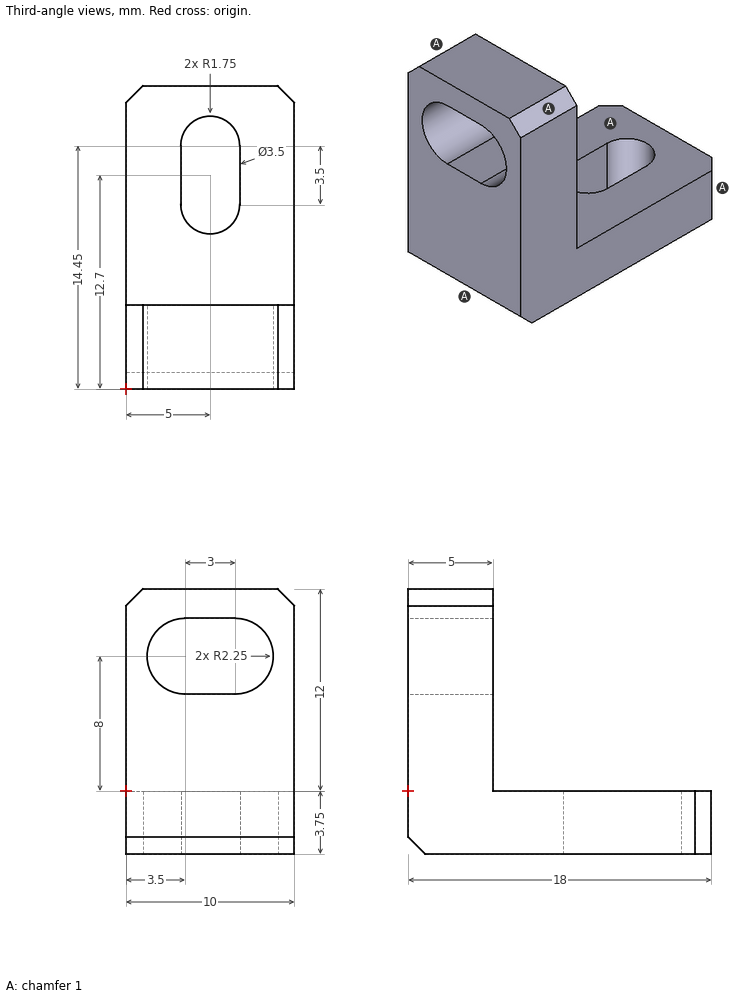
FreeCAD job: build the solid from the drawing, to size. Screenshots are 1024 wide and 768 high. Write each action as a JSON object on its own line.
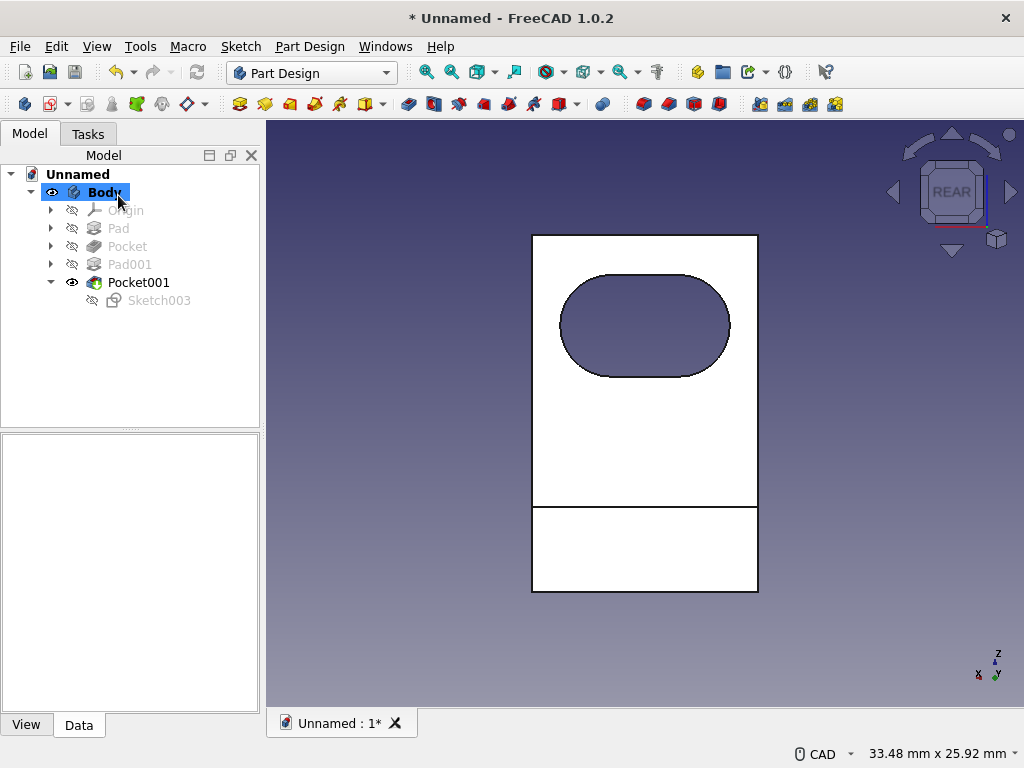
{"action": "left_click", "coordinate": [758, 548]}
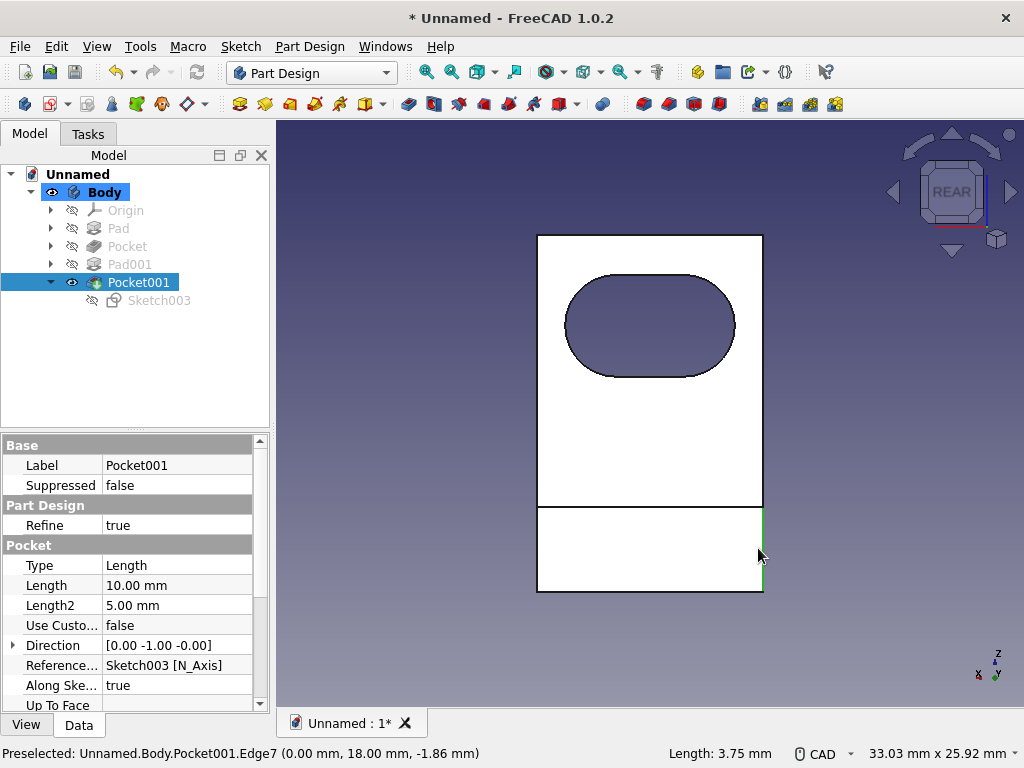
{"action": "key", "text": "0"}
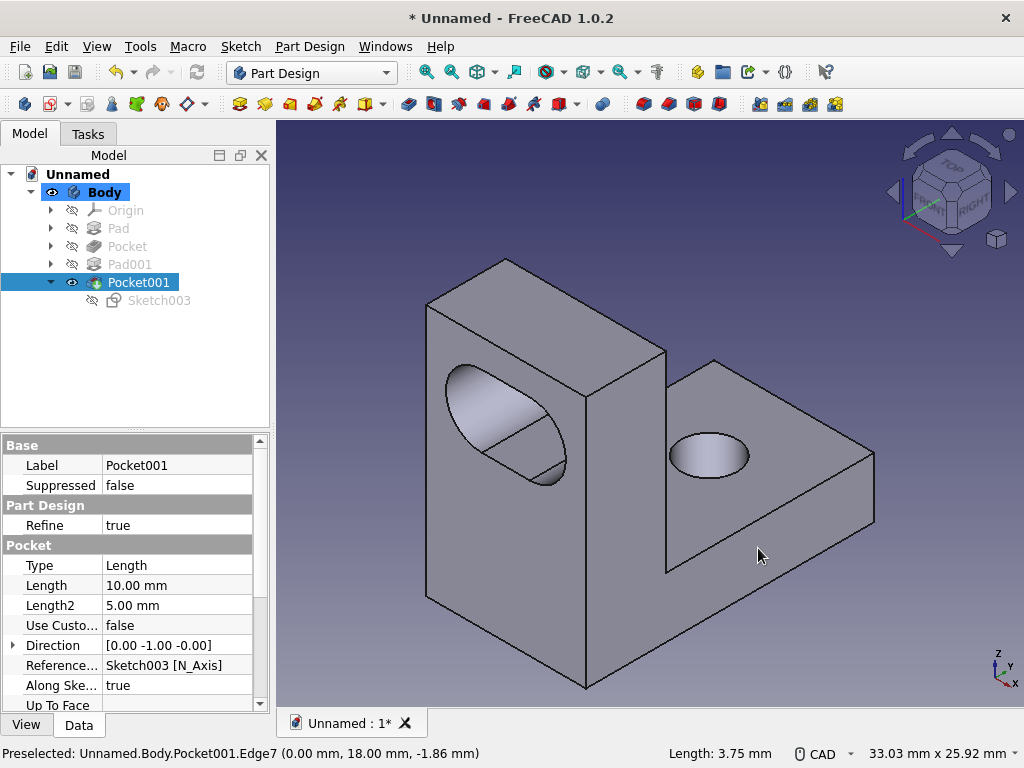
{"action": "left_click", "coordinate": [626, 373], "text": "ctrl"}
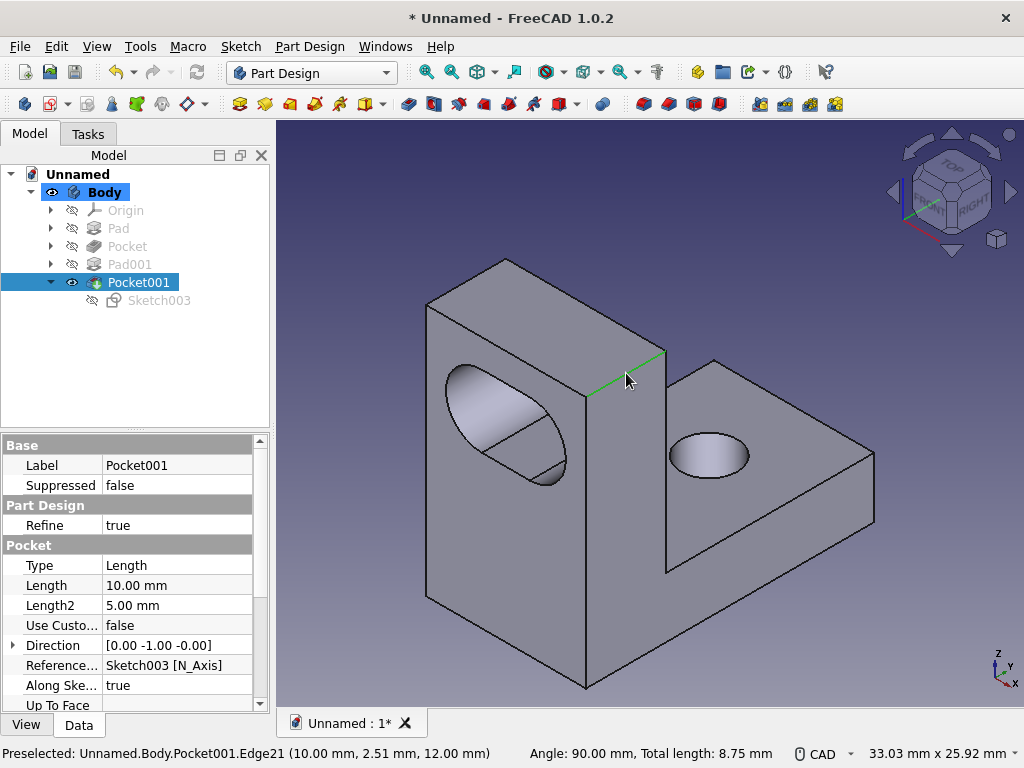
{"action": "key", "text": "2"}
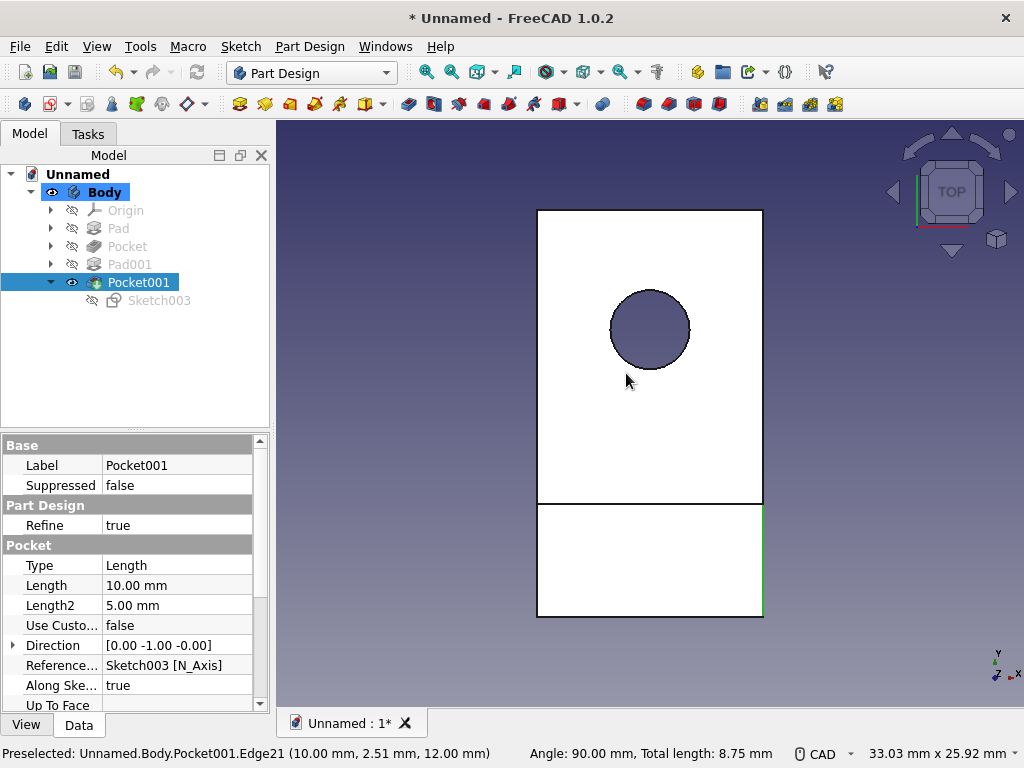
{"action": "left_click", "coordinate": [537, 560], "text": "ctrl"}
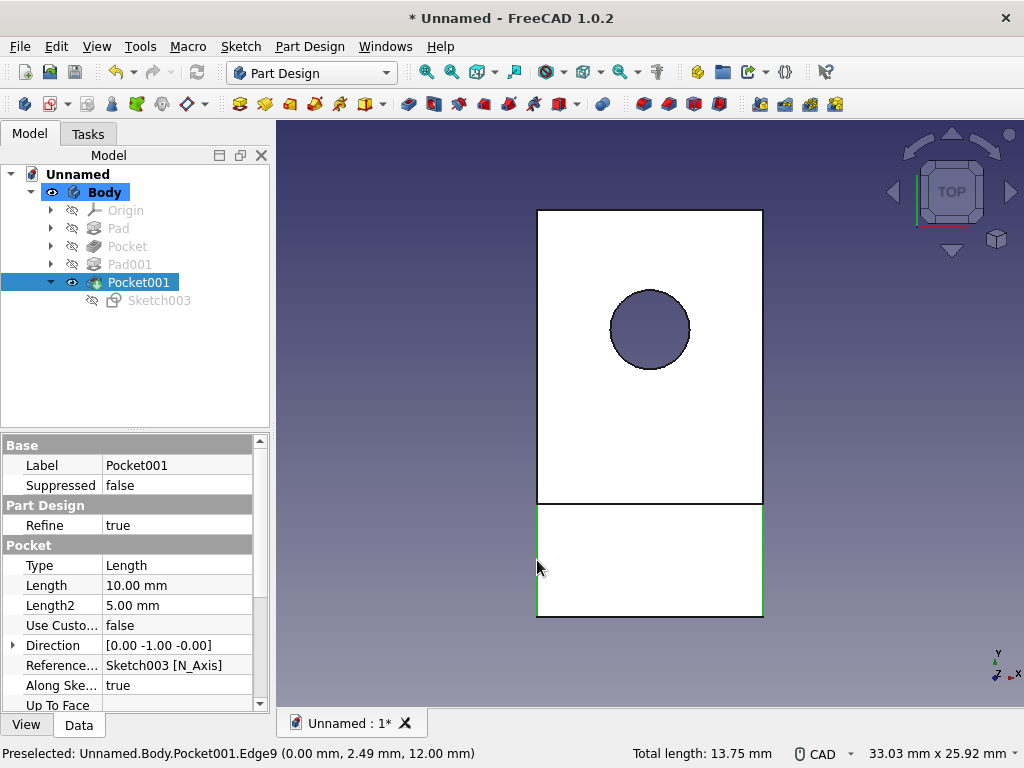
{"action": "key", "text": "1"}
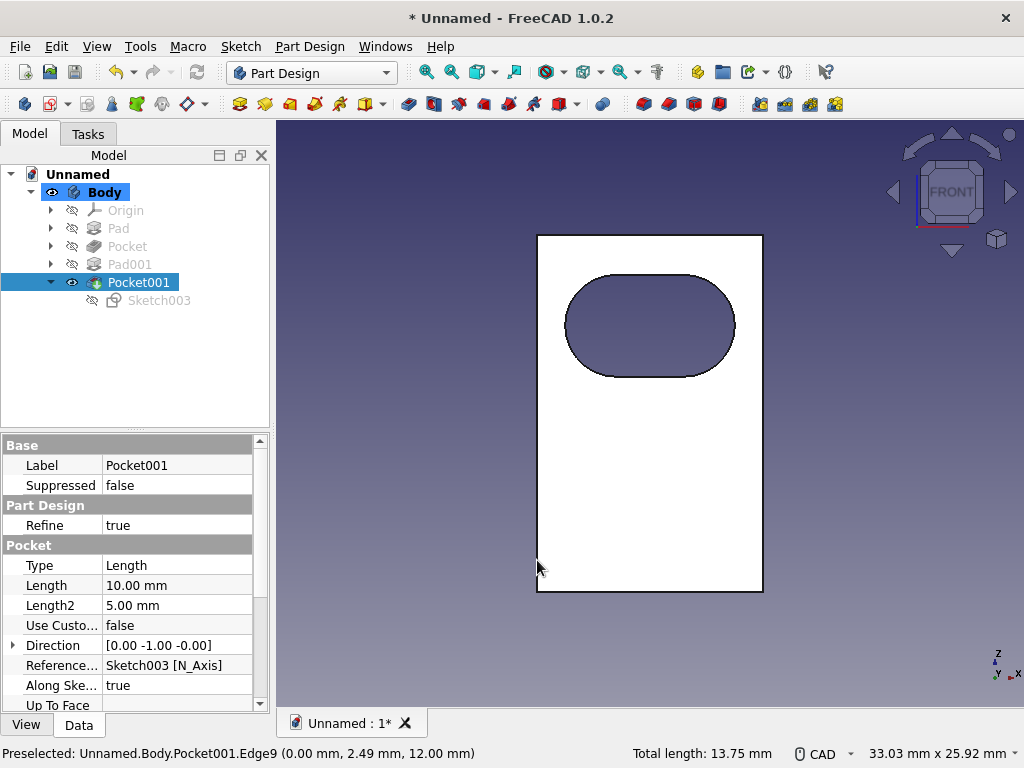
{"action": "key", "text": "3"}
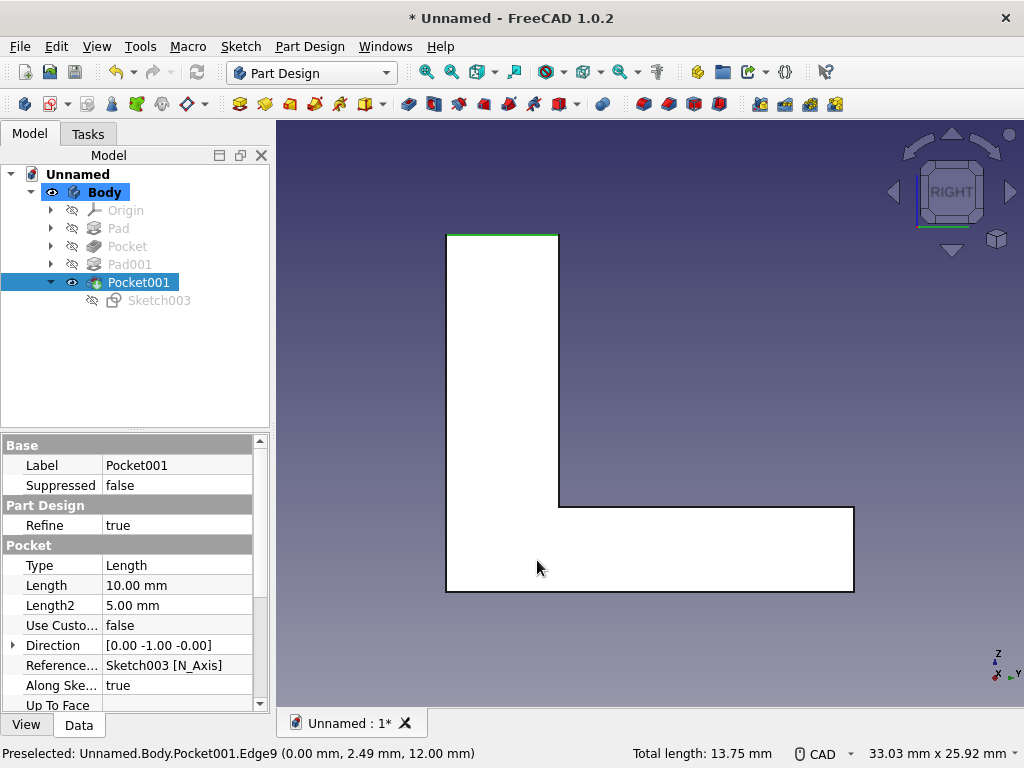
{"action": "left_click", "coordinate": [854, 548], "text": "ctrl"}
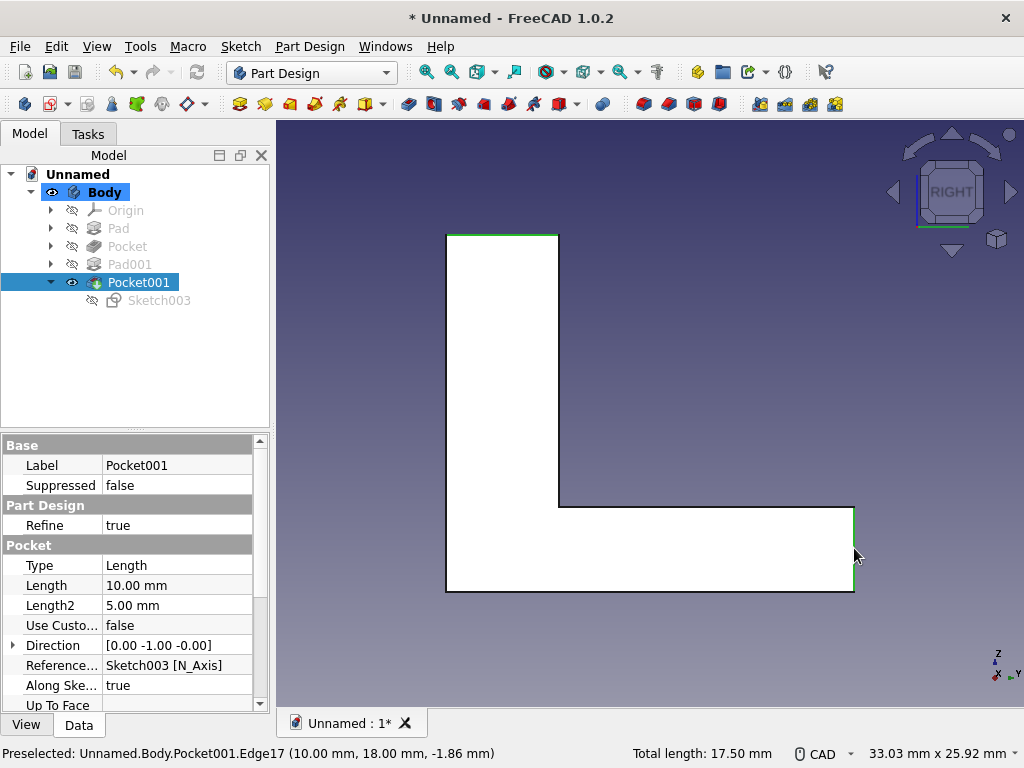
{"action": "key", "text": "5"}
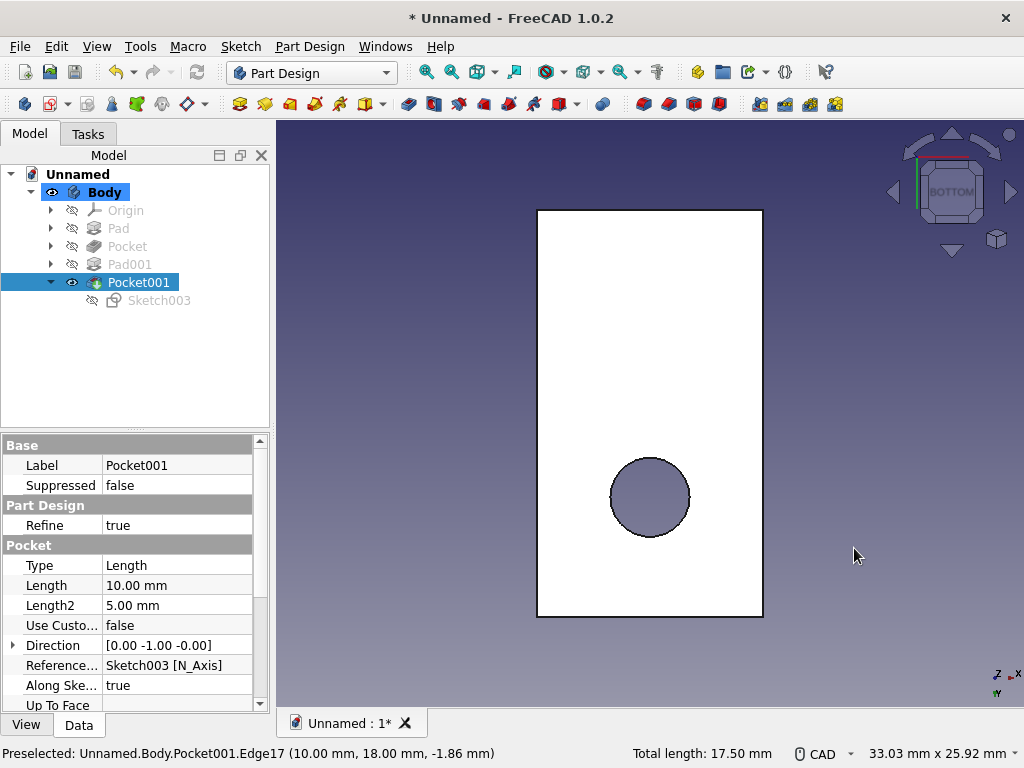
{"action": "left_click", "coordinate": [650, 209], "text": "ctrl"}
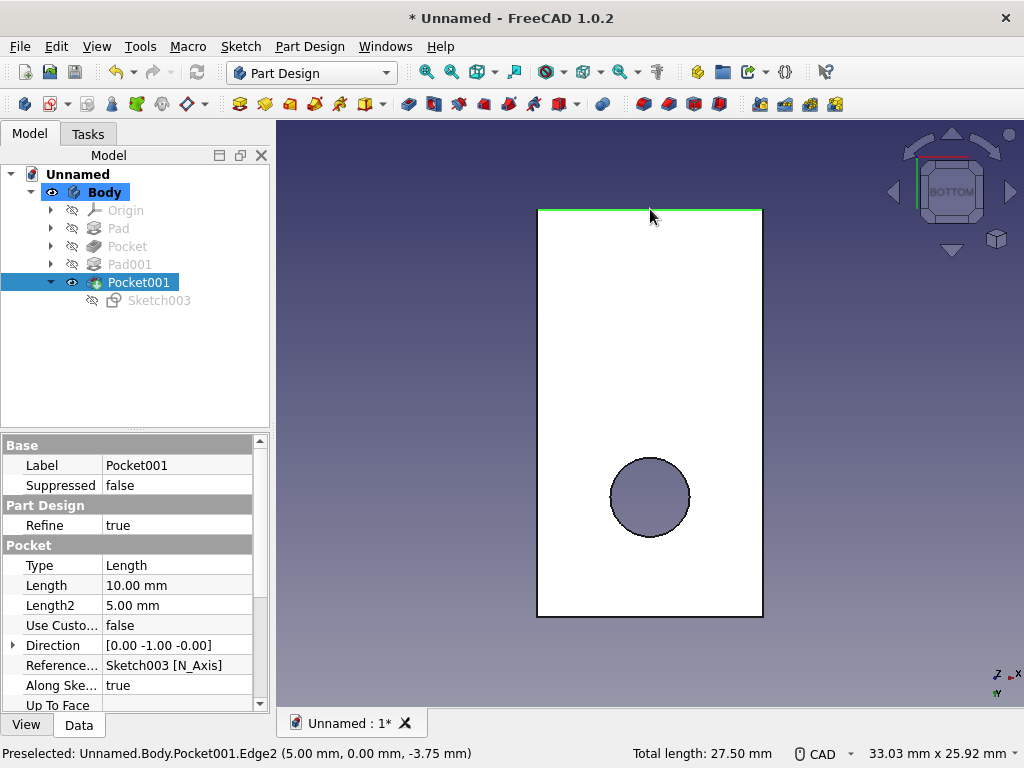
{"action": "left_click", "coordinate": [669, 104]}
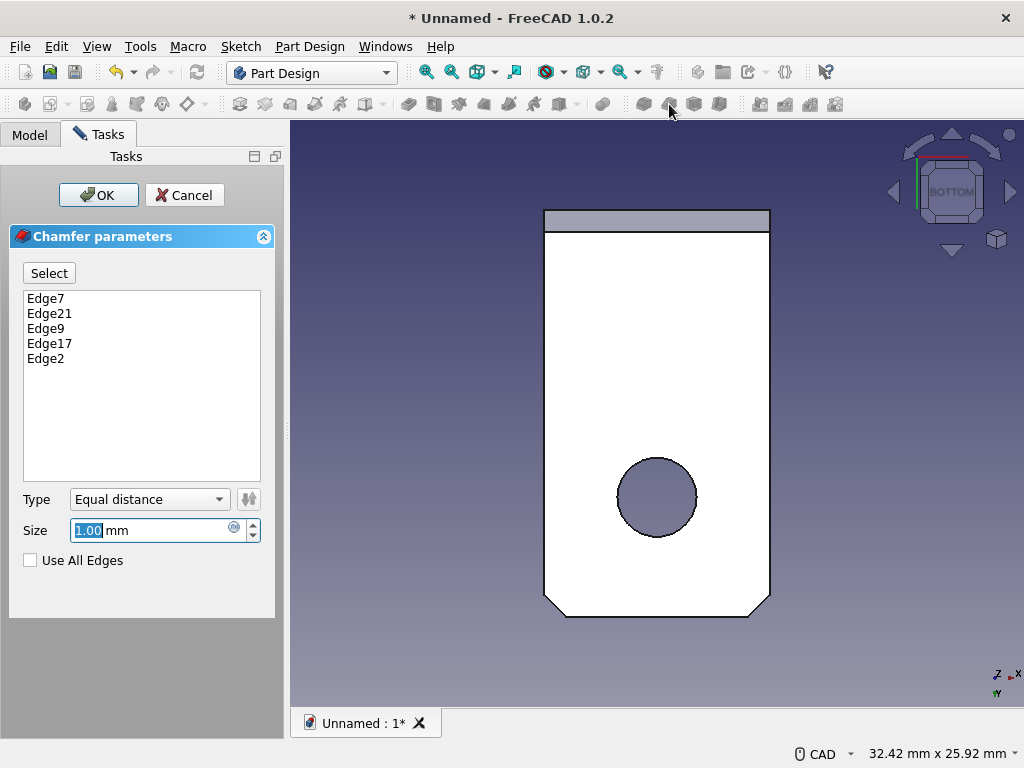
{"action": "type", "text": "1"}
{"action": "key", "text": "Tab"}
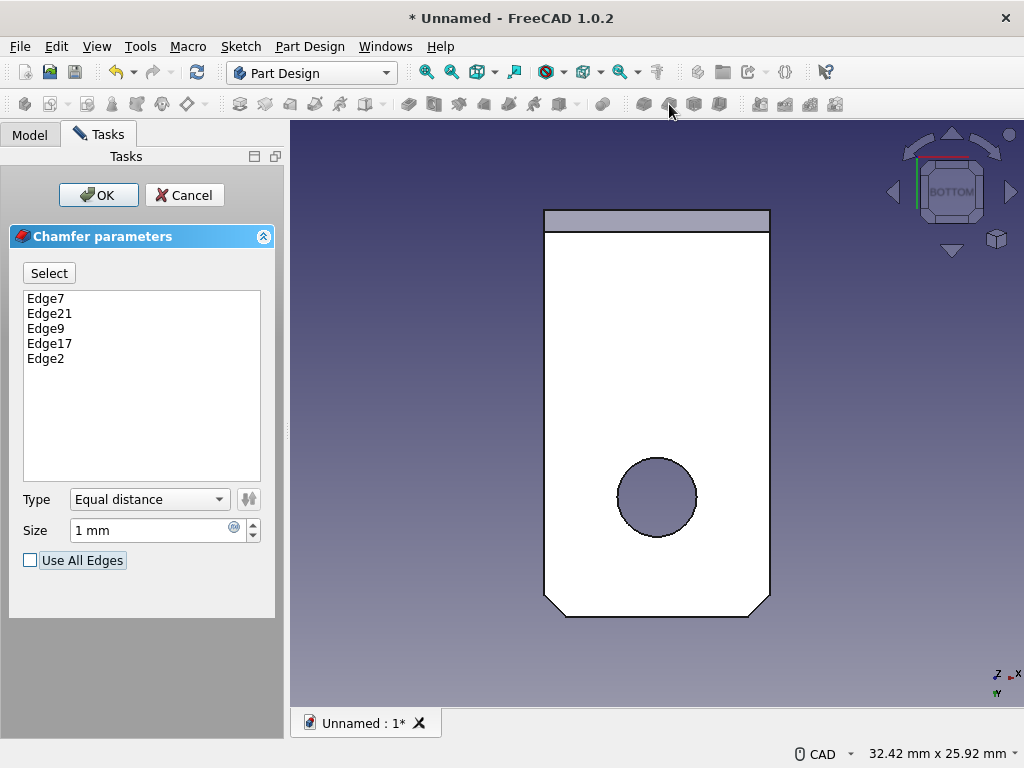
{"action": "left_click", "coordinate": [99, 195]}